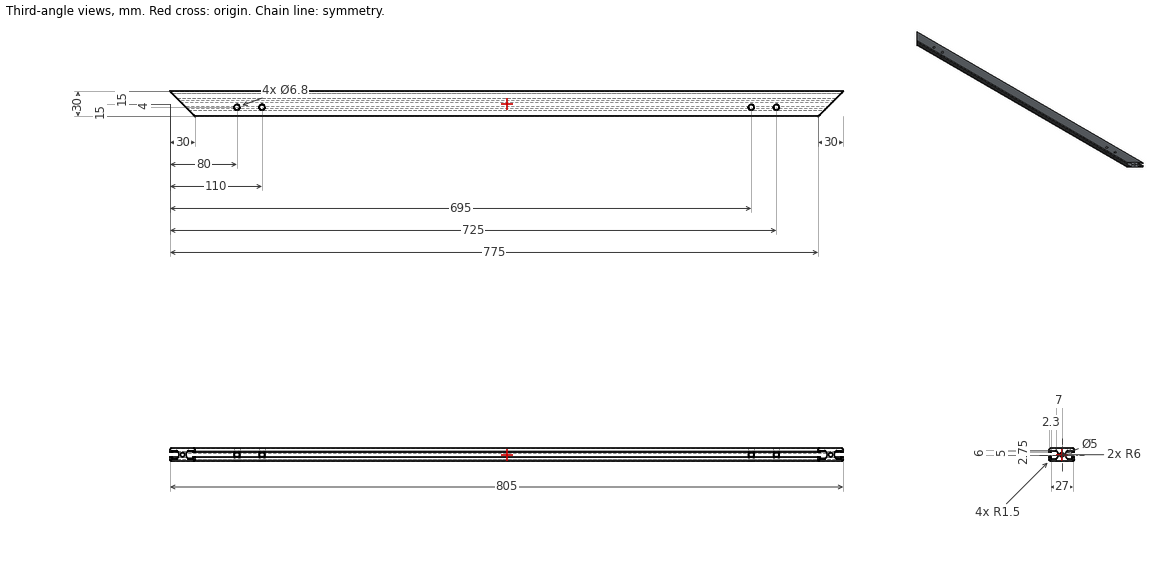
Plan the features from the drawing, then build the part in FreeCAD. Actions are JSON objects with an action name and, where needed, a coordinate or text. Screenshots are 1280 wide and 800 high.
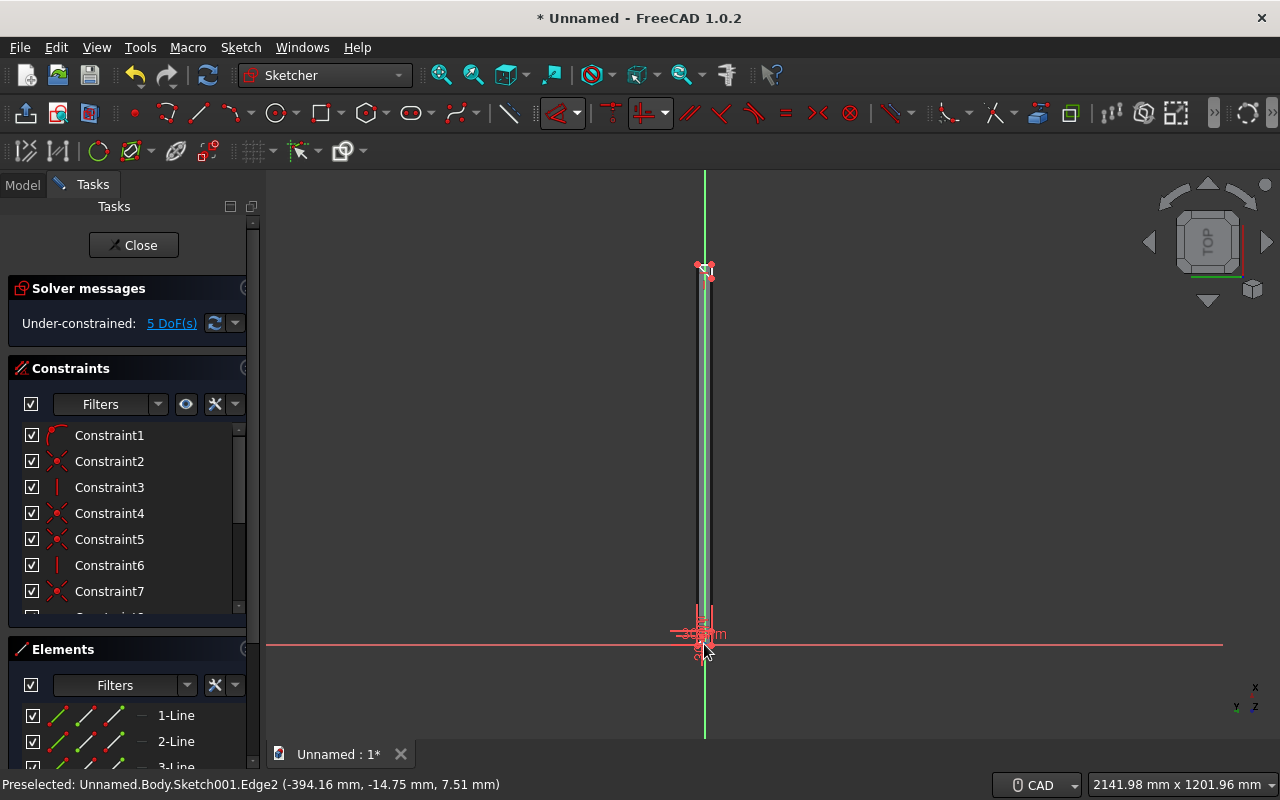
{"action": "scroll", "coordinate": [712, 275], "scroll_direction": "up", "scroll_amount": 8}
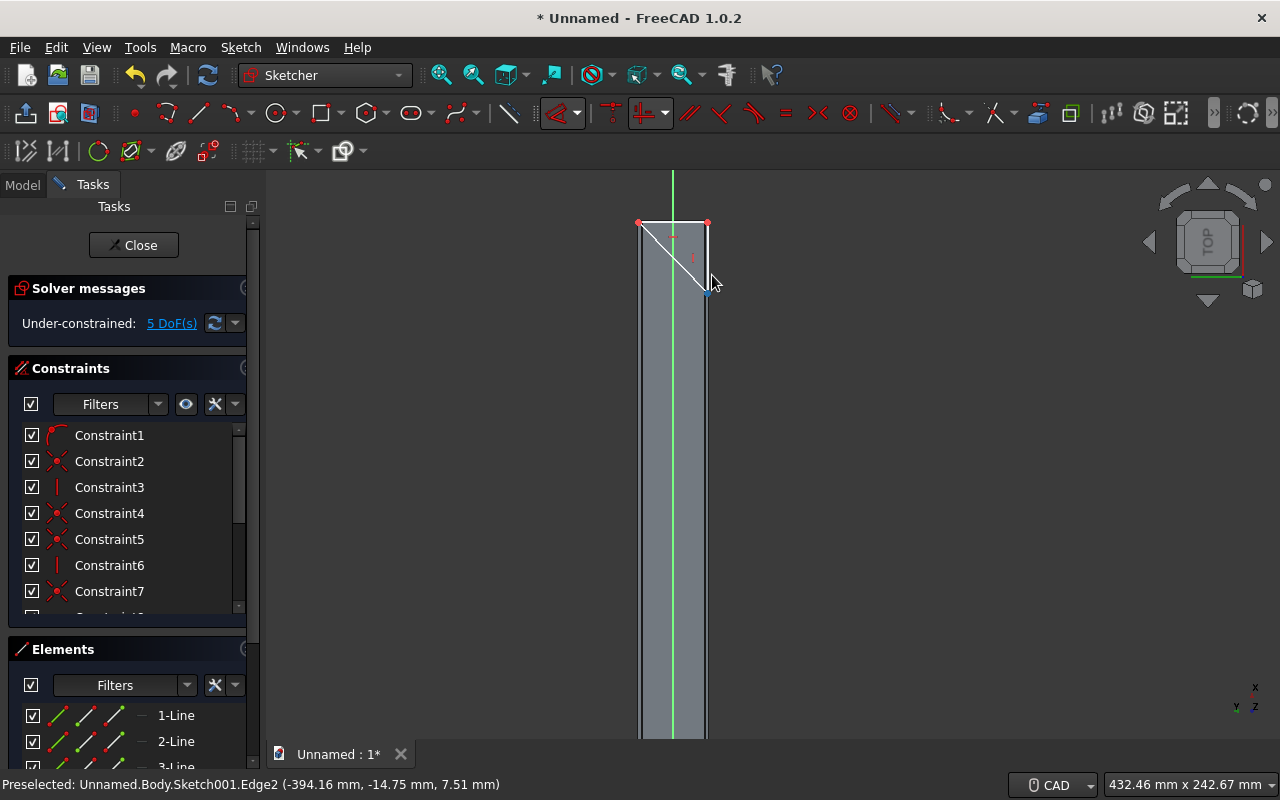
{"action": "left_click", "coordinate": [708, 272]}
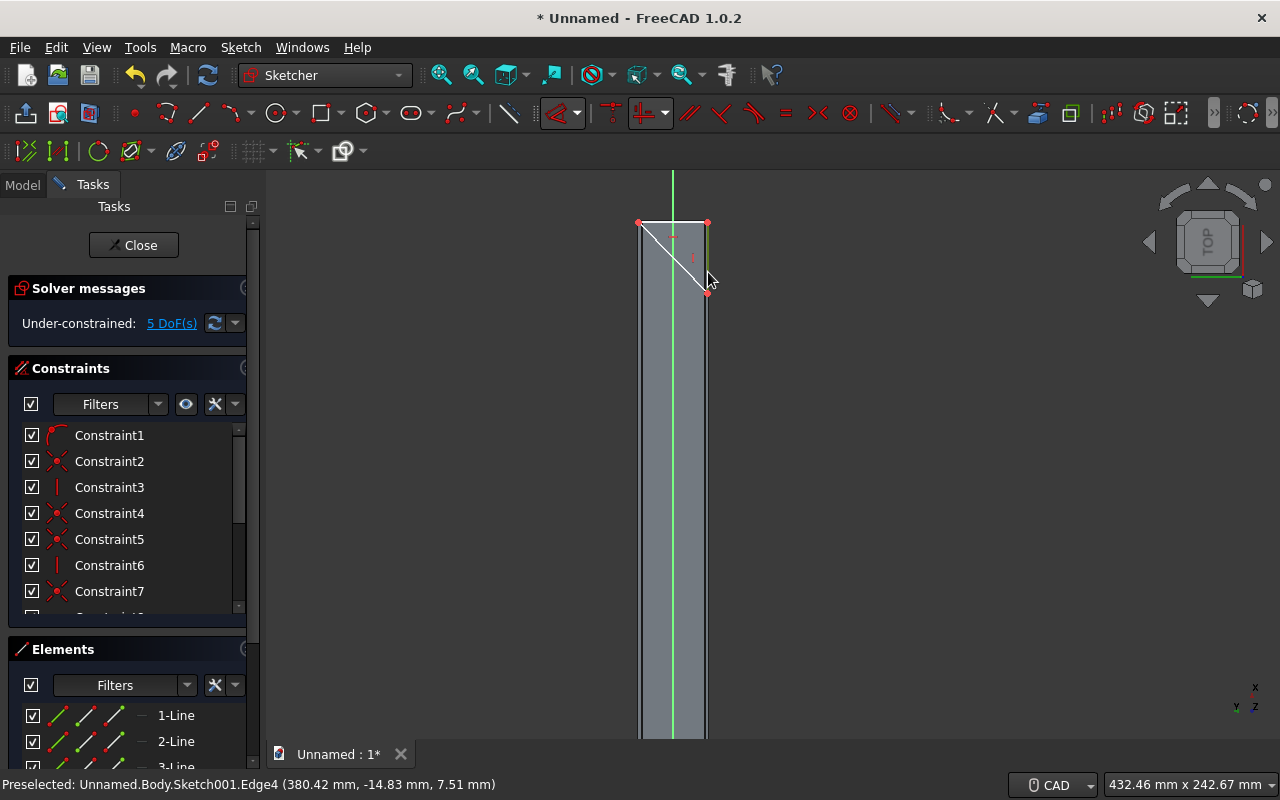
{"action": "left_click", "coordinate": [580, 114]}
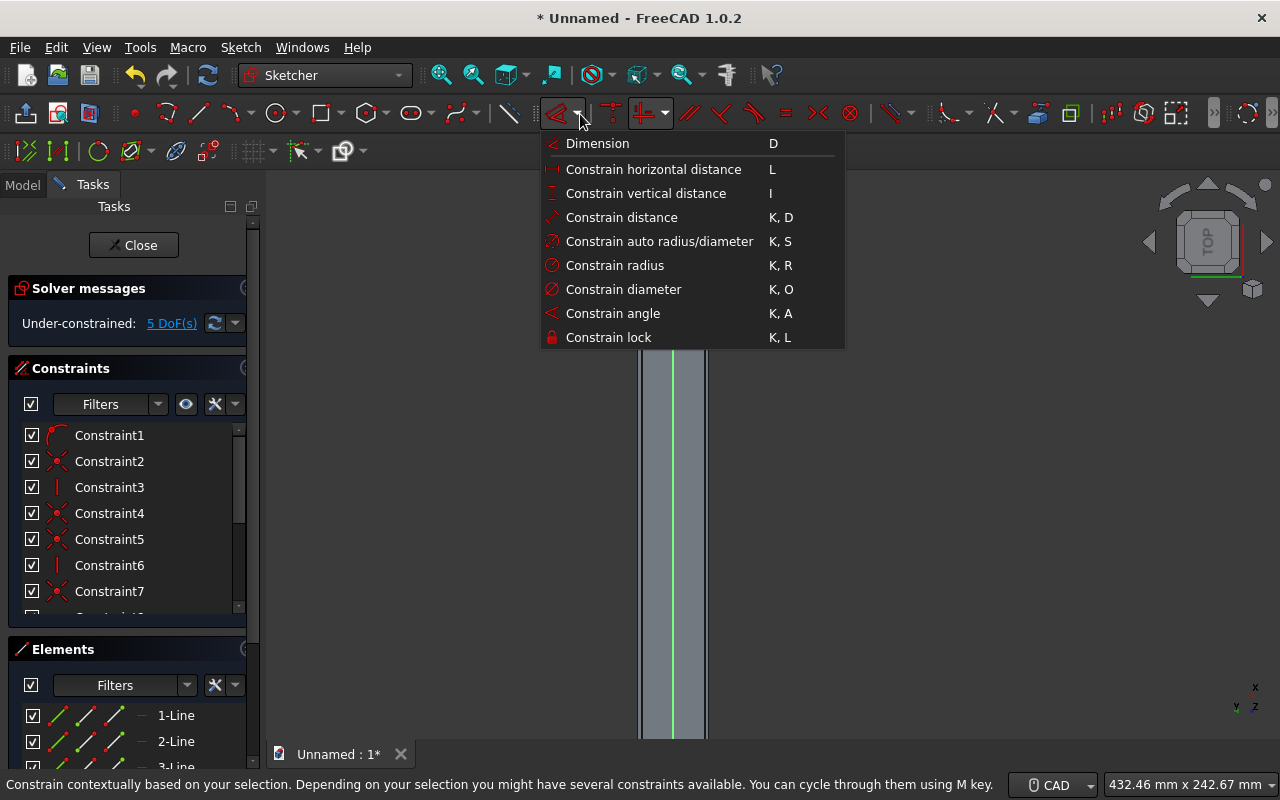
{"action": "left_click", "coordinate": [693, 193]}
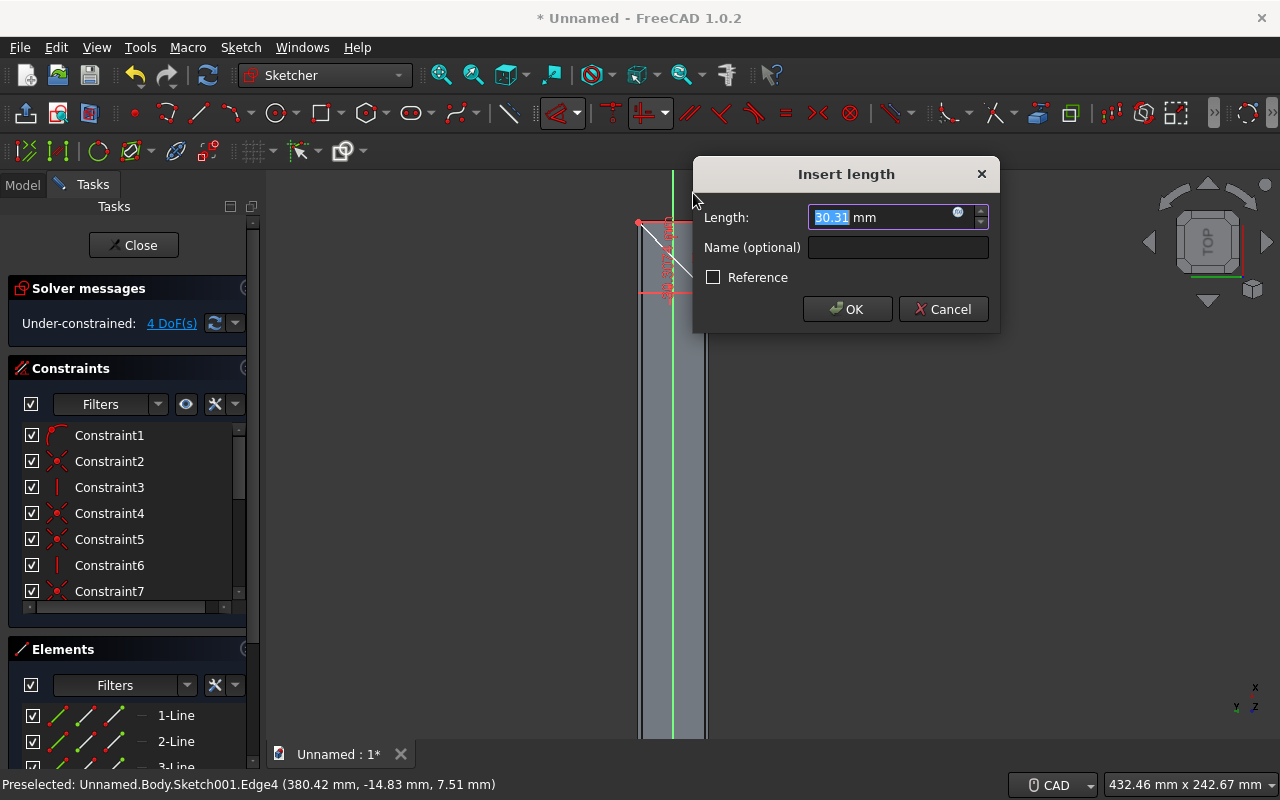
{"action": "type", "text": "30"}
{"action": "key", "text": "Return"}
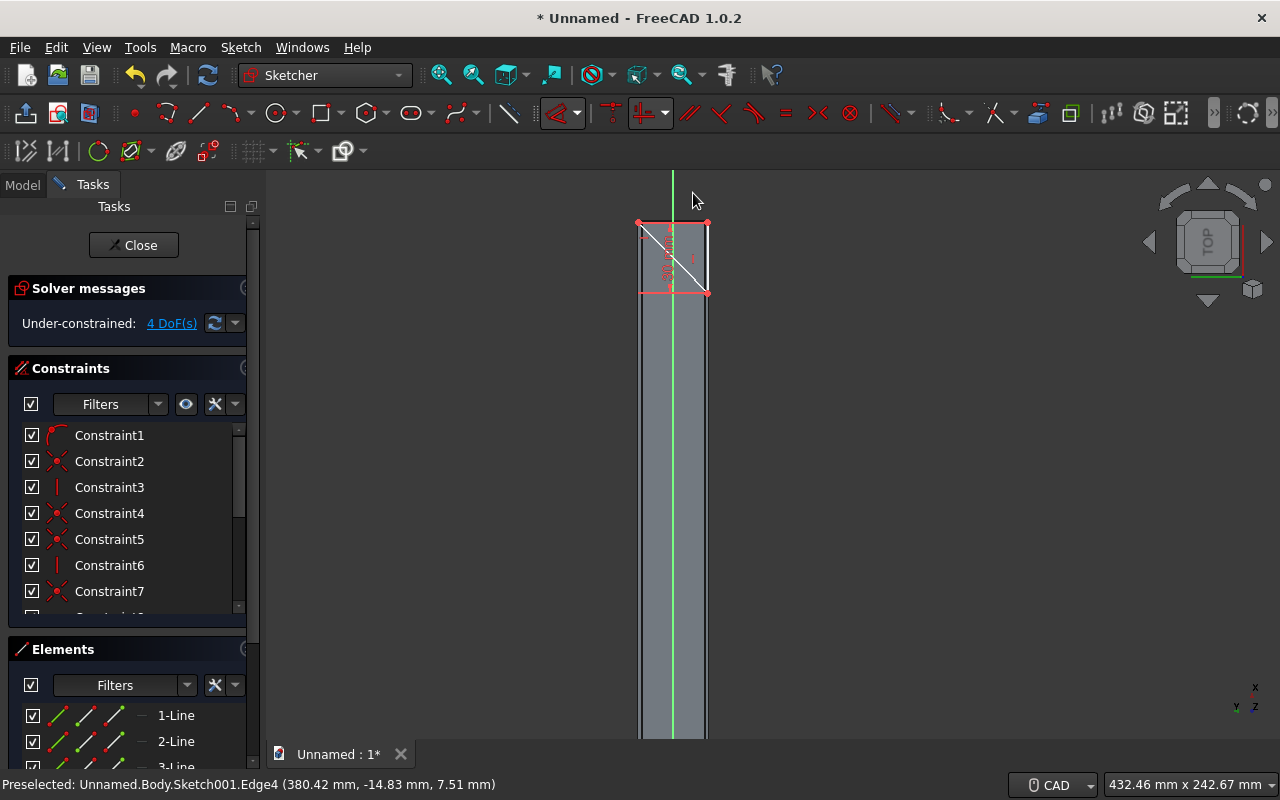
{"action": "left_click", "coordinate": [687, 223]}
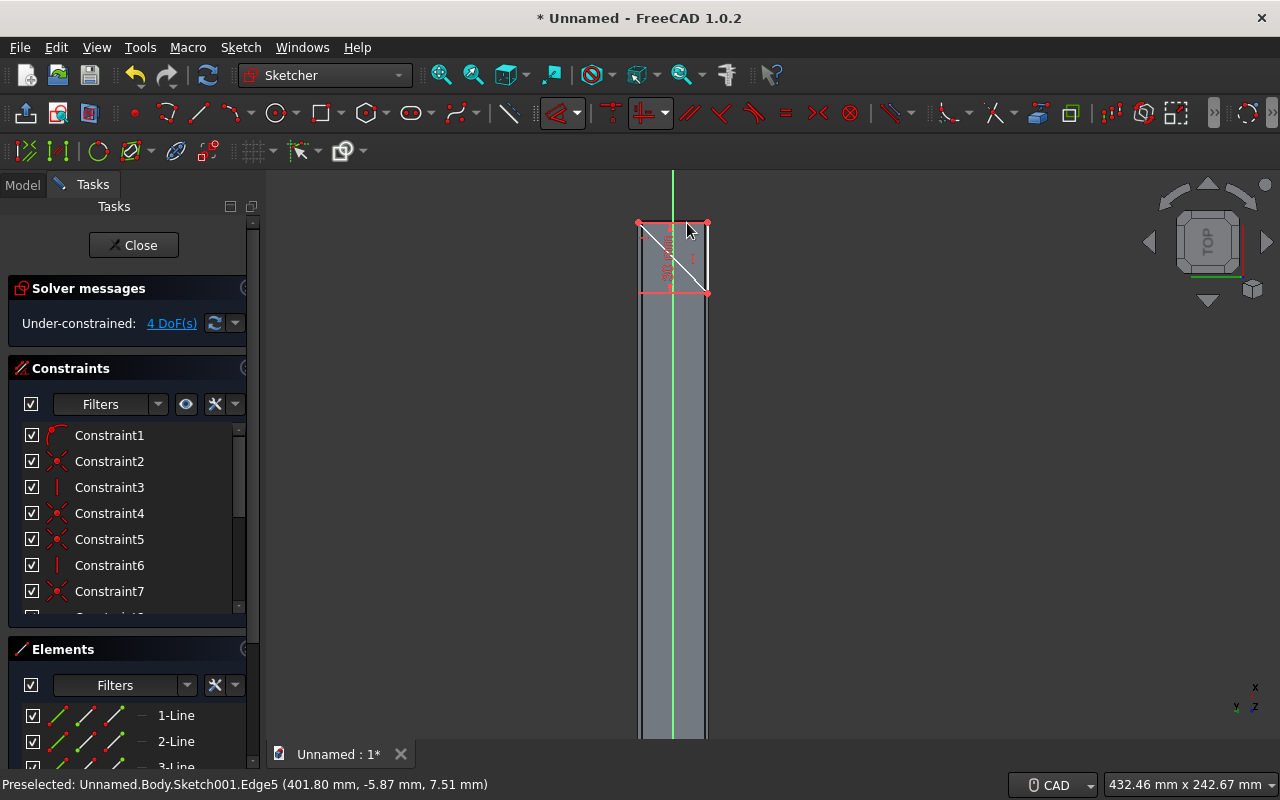
{"action": "key", "text": "l"}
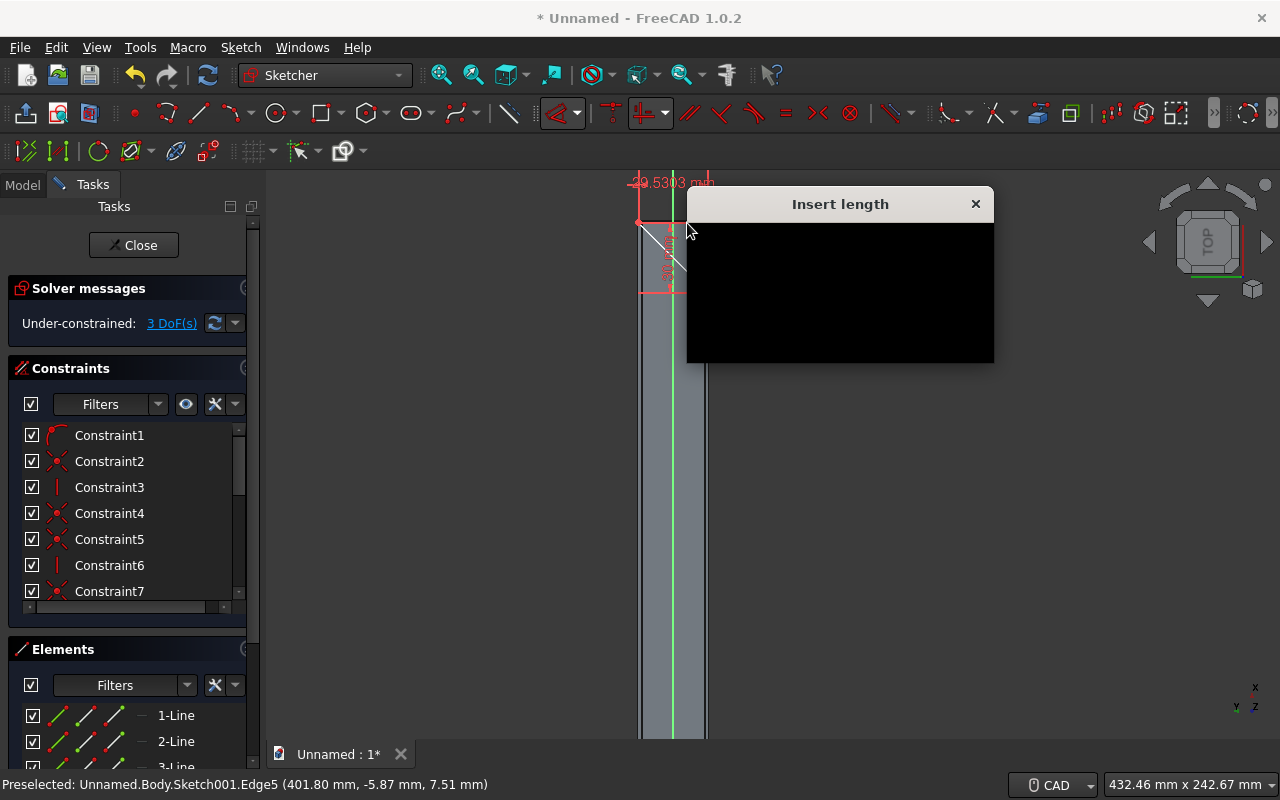
{"action": "type", "text": "30"}
{"action": "key", "text": "Return"}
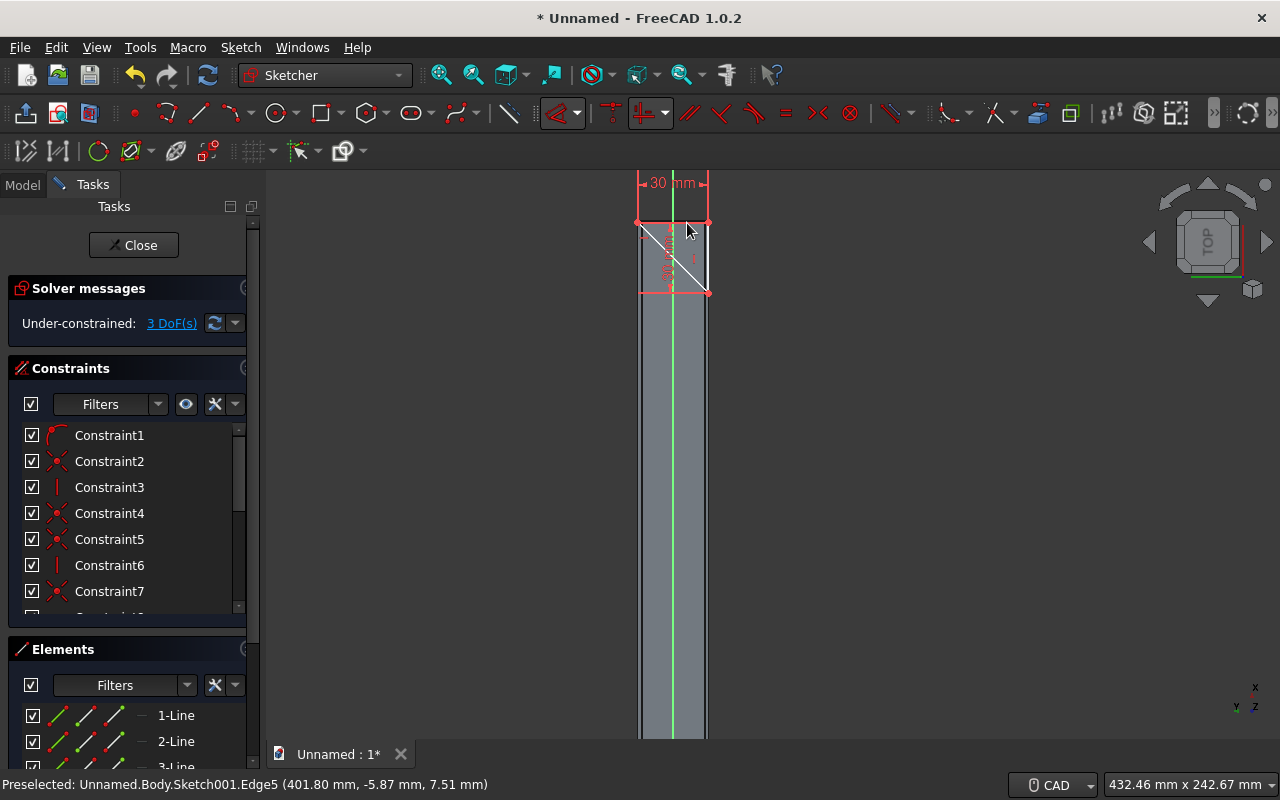
{"action": "scroll", "coordinate": [712, 275], "scroll_direction": "down", "scroll_amount": 8}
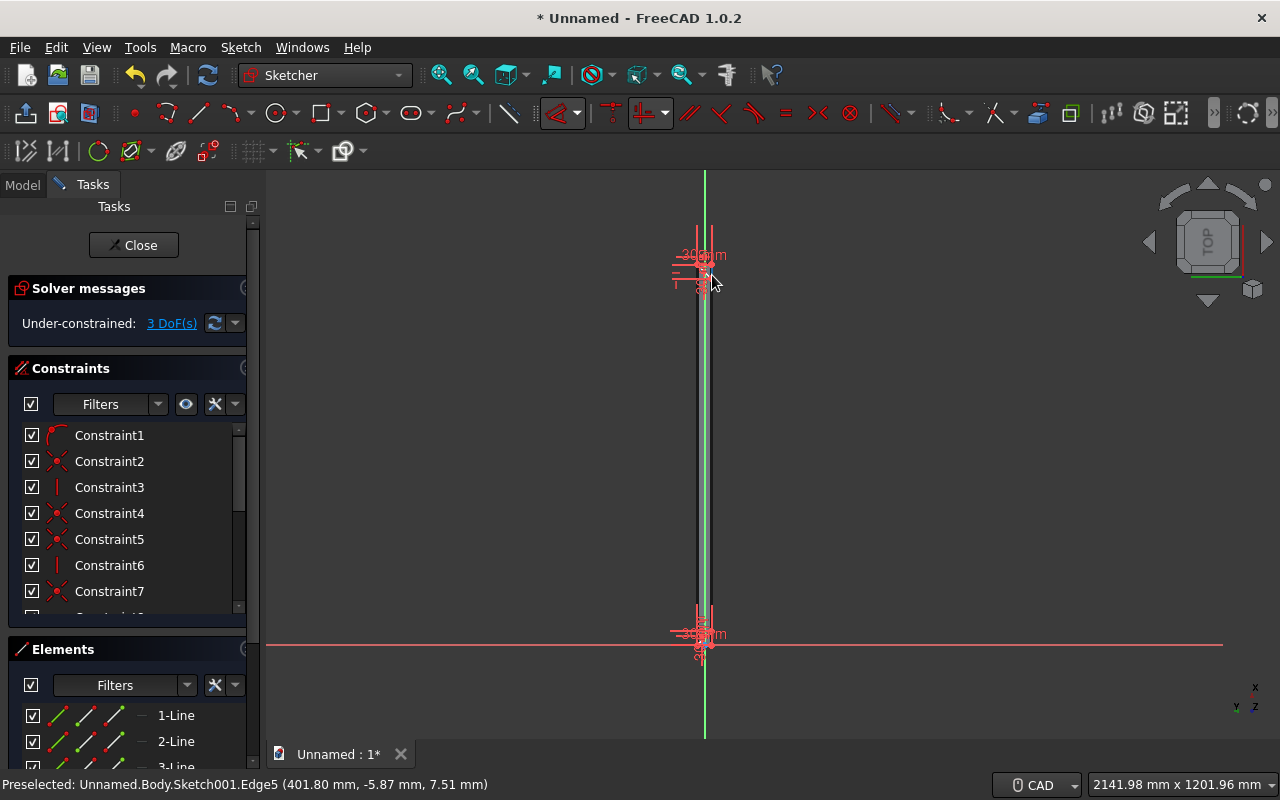
{"action": "scroll", "coordinate": [697, 645], "scroll_direction": "up", "scroll_amount": 9}